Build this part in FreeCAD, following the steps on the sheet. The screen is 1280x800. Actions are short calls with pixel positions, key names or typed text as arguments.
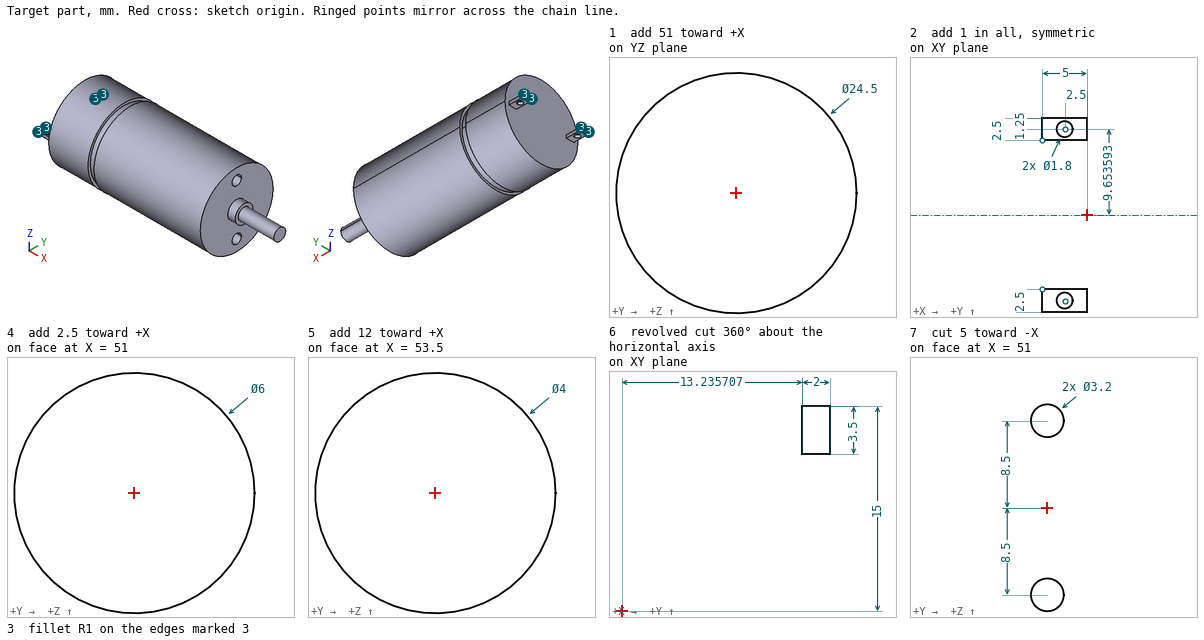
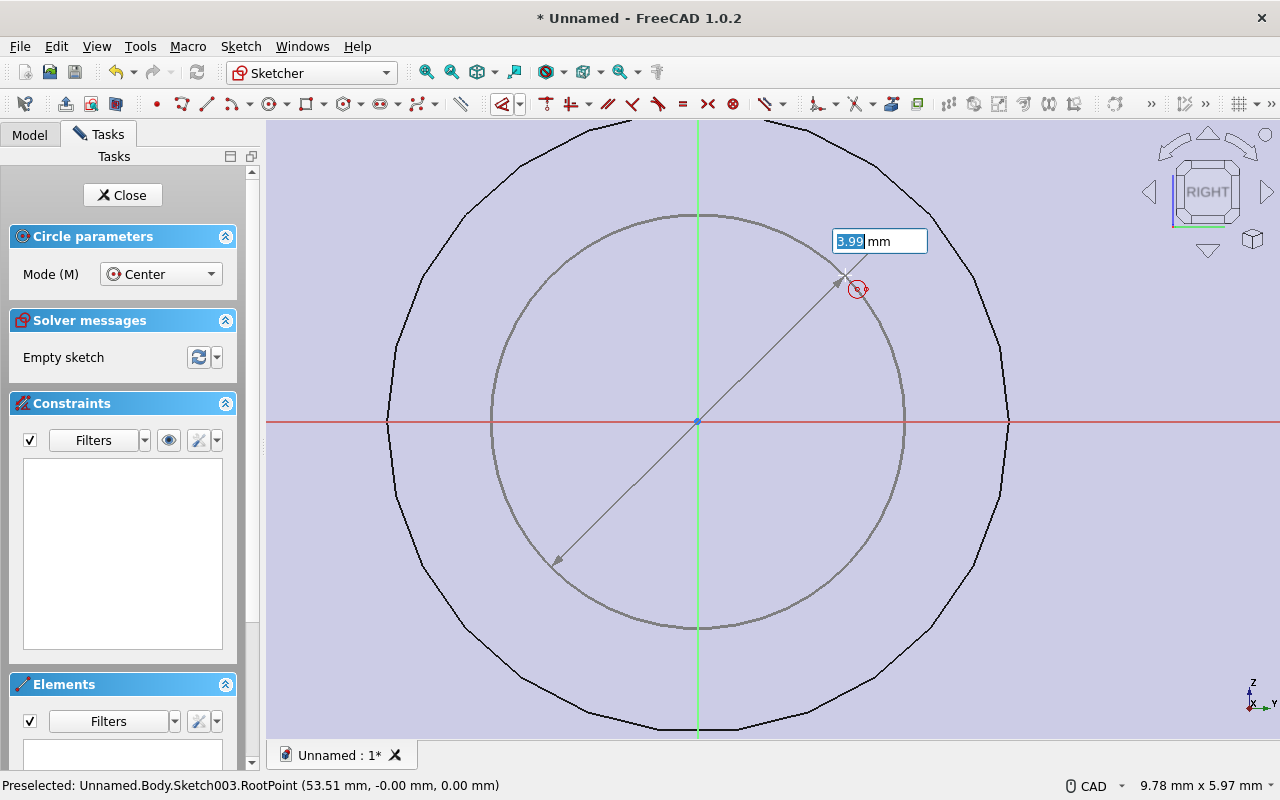
text(4)
key(Return)
key(Escape)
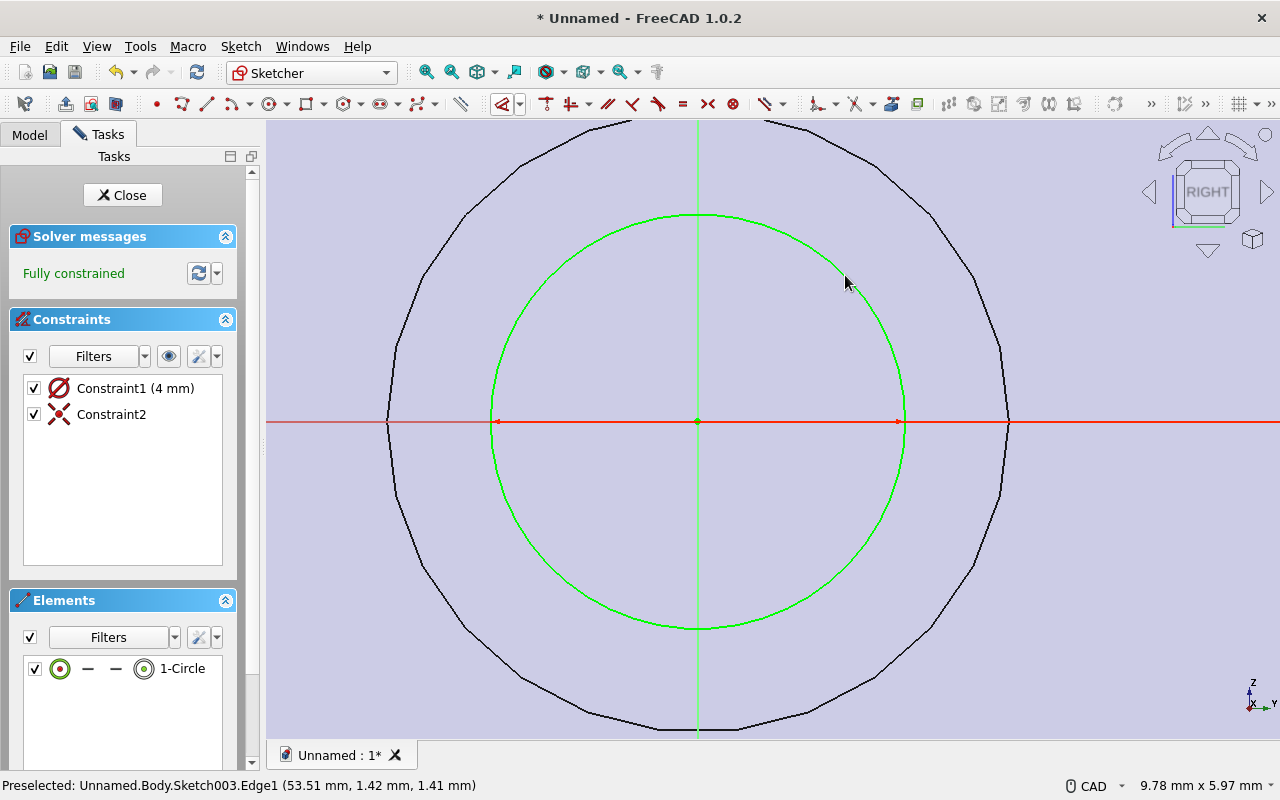
click(123, 195)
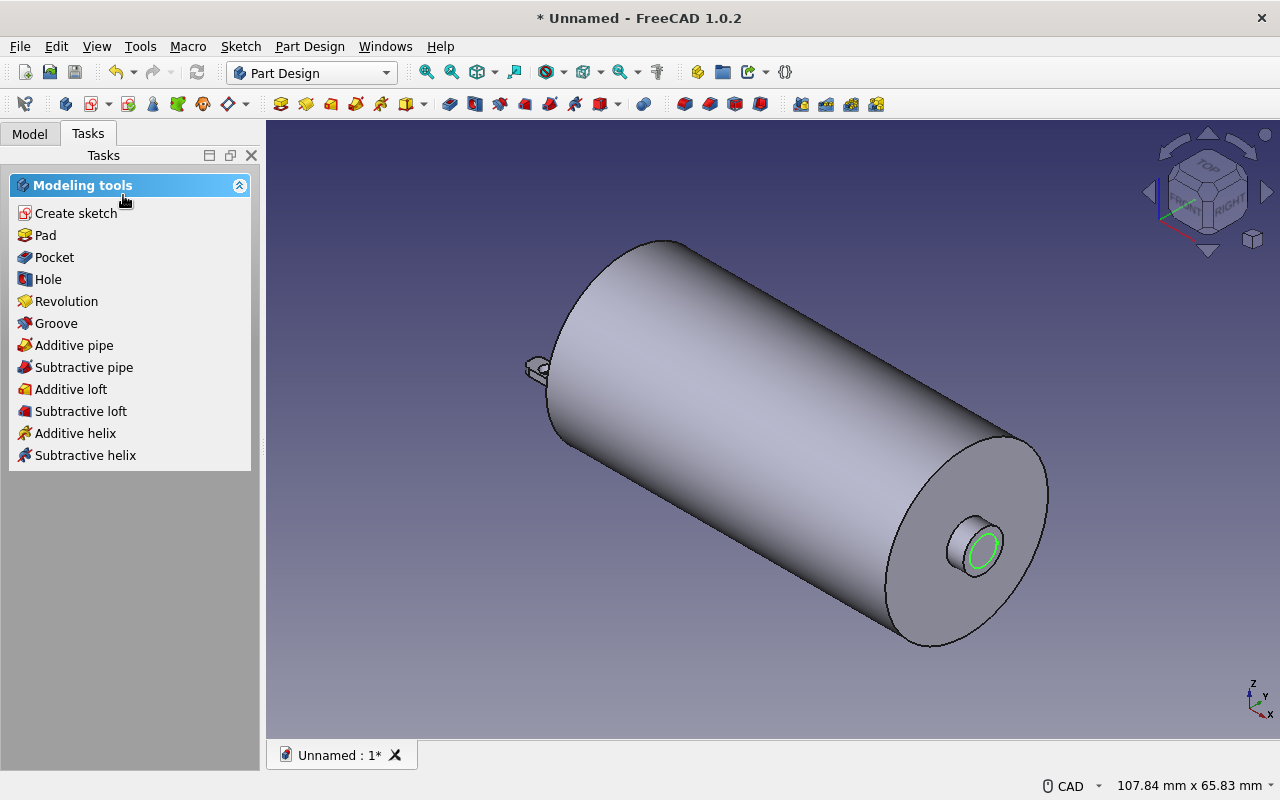
click(281, 104)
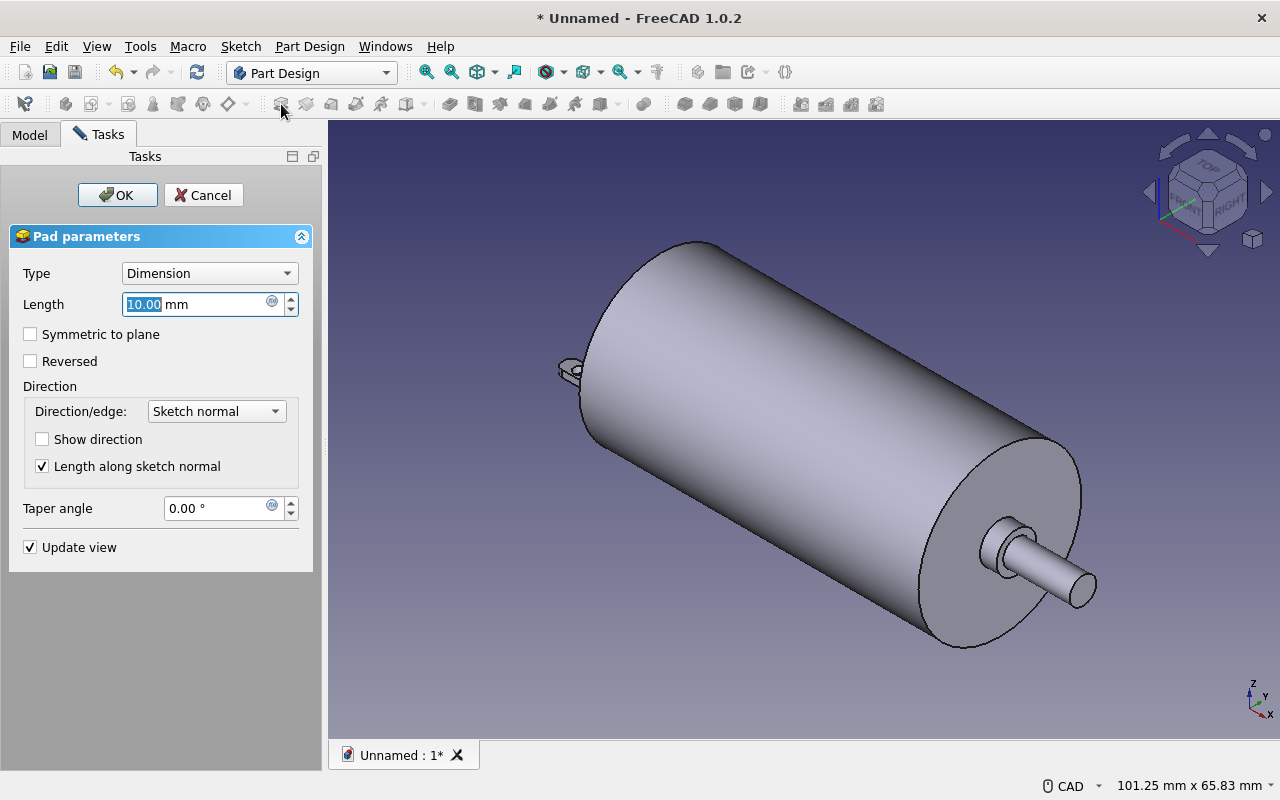
text(12)
key(Tab)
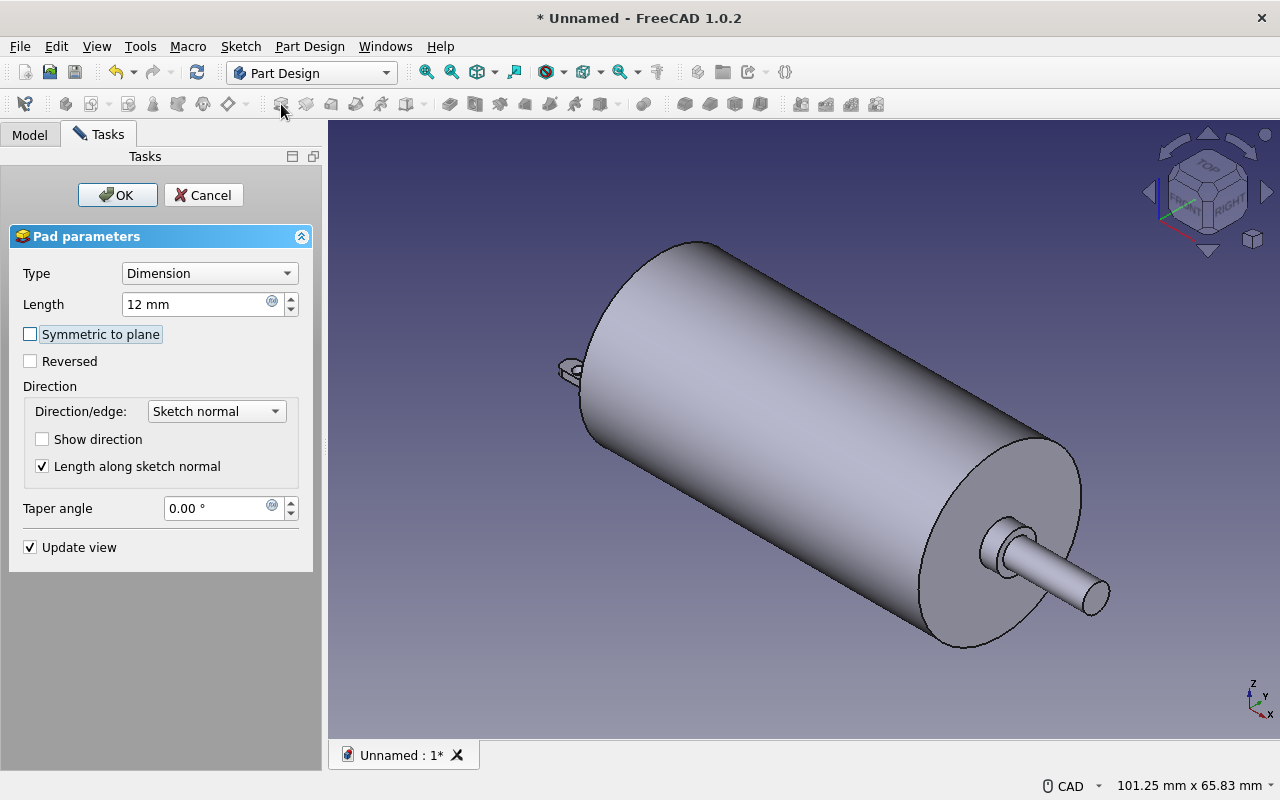
click(118, 195)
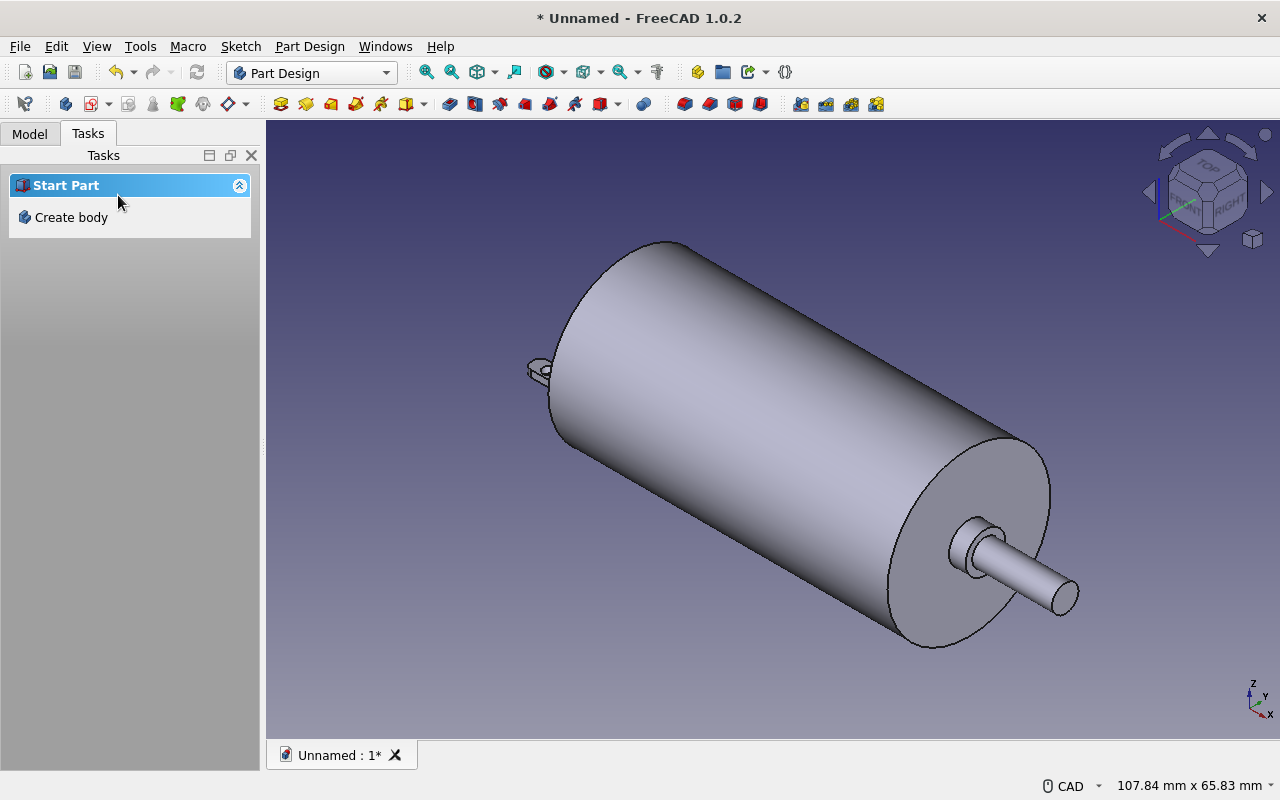
click(90, 104)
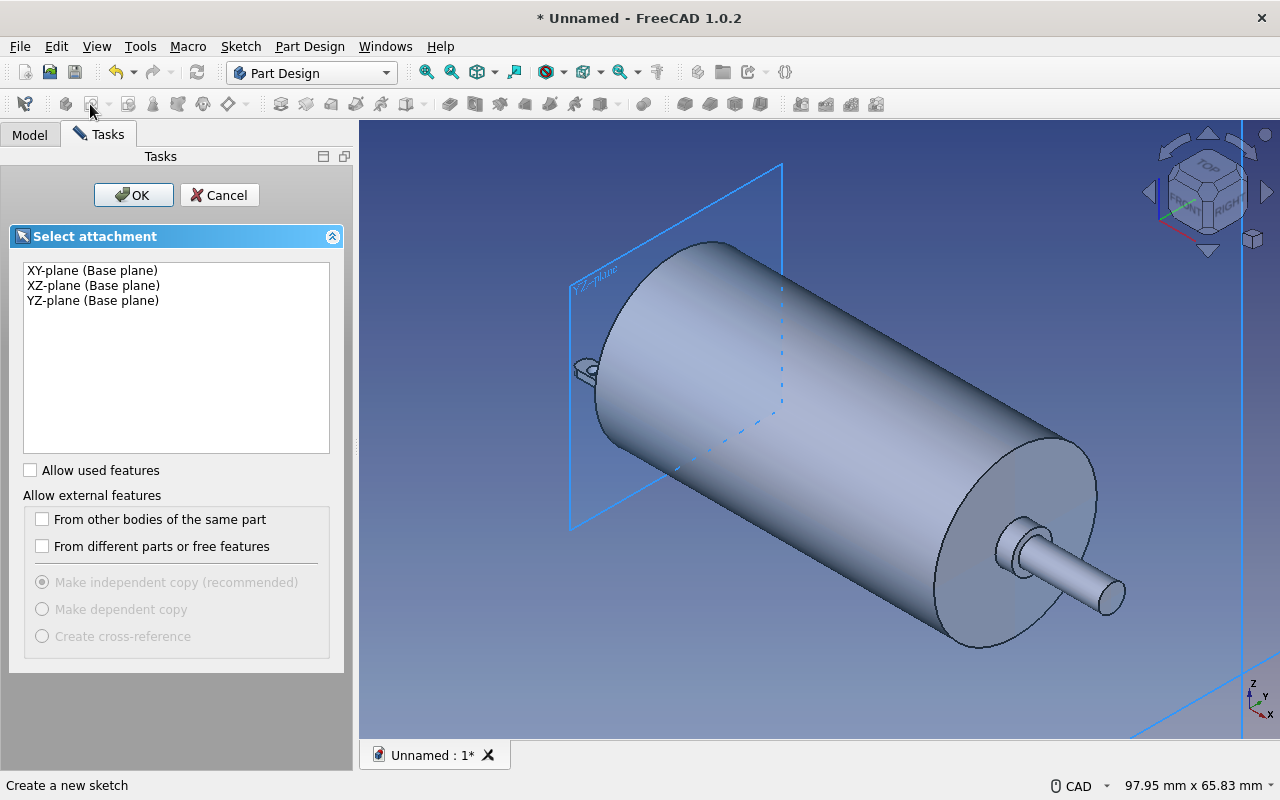
click(84, 270)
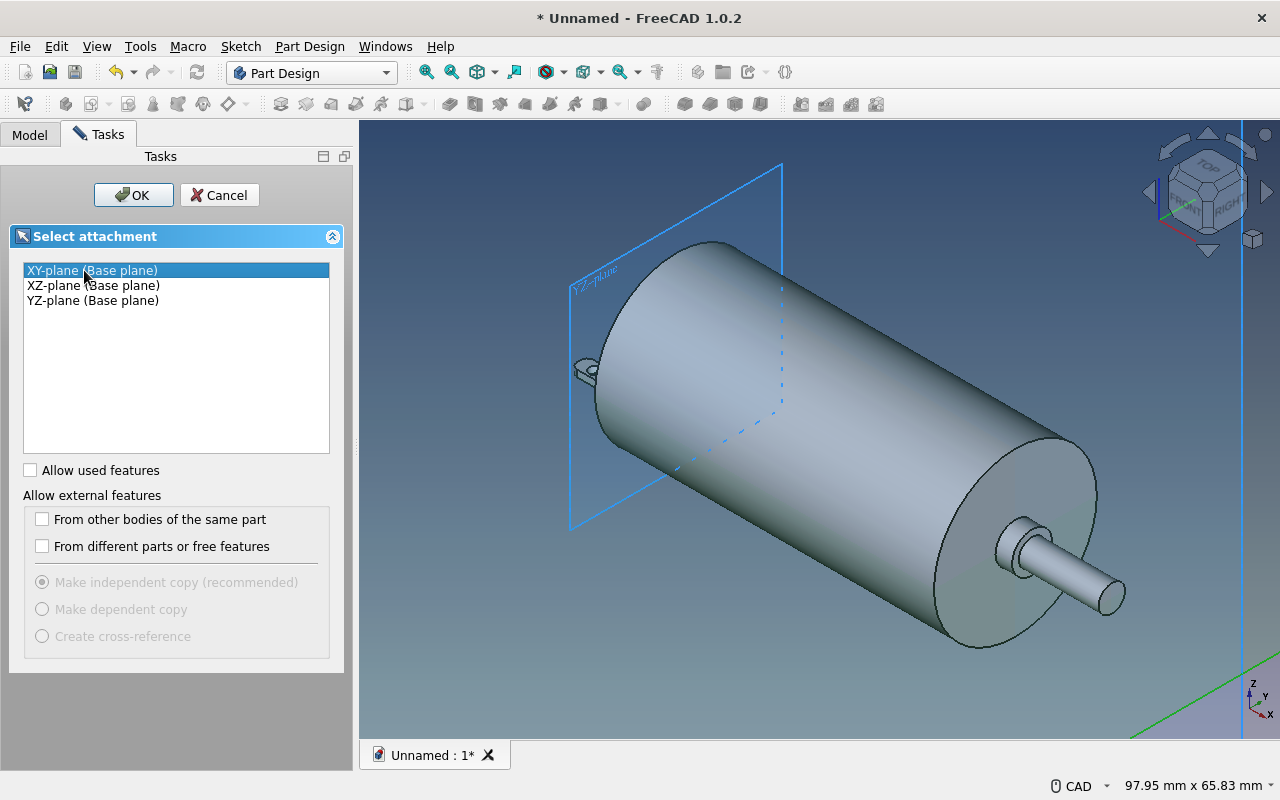
click(134, 195)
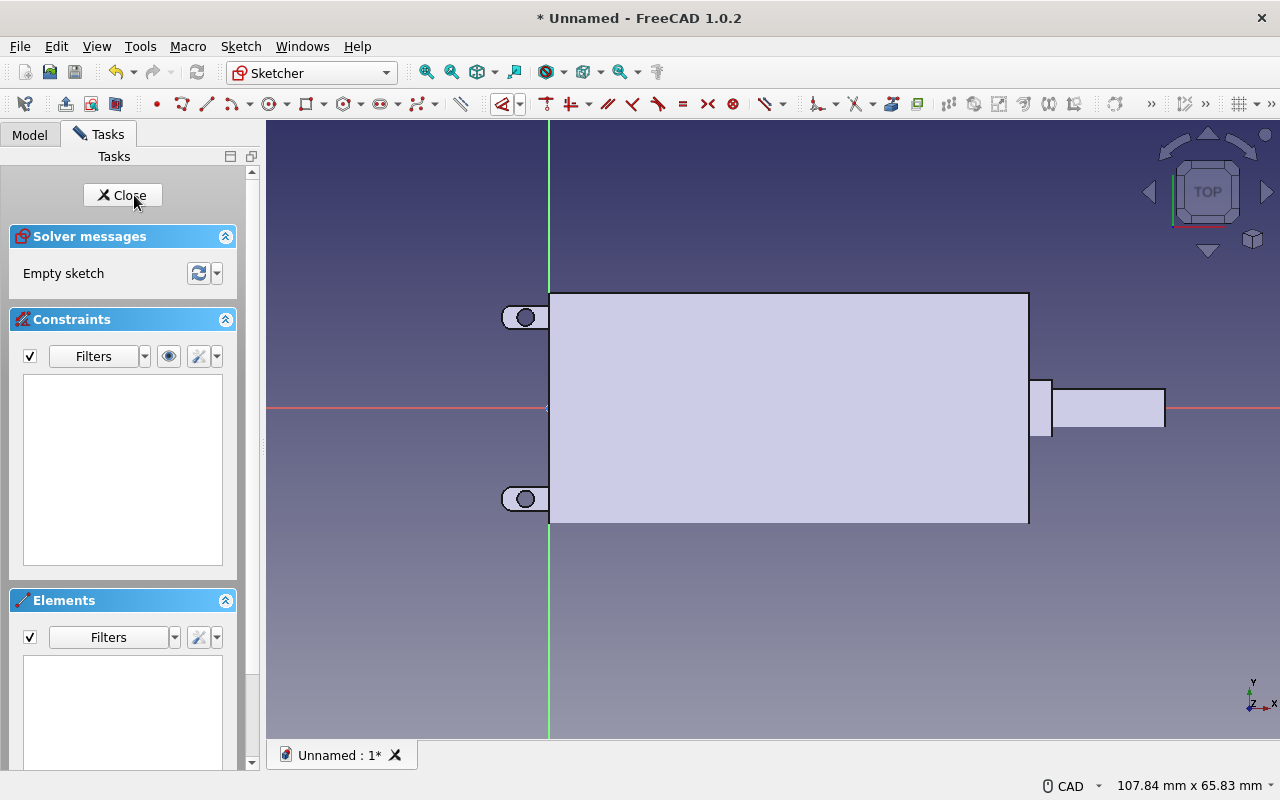
click(116, 104)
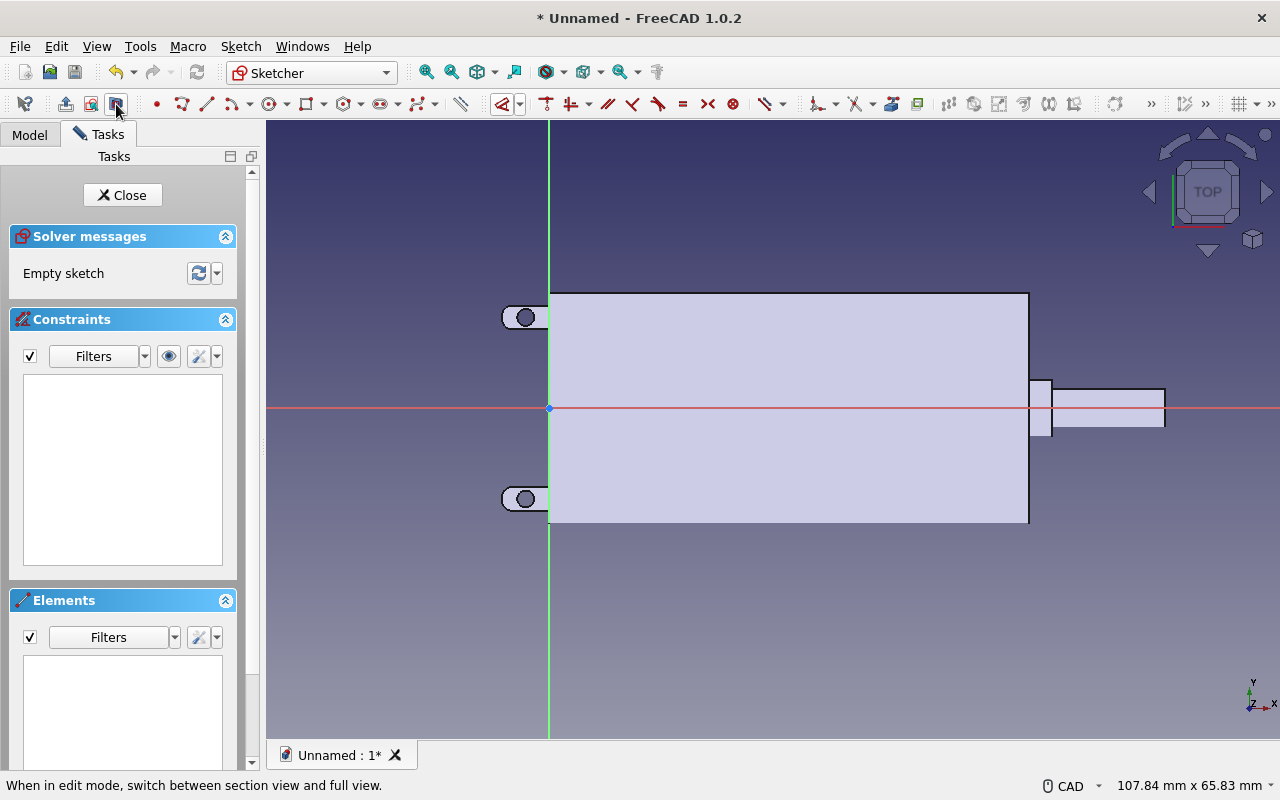
scroll(681, 269, up, 12)